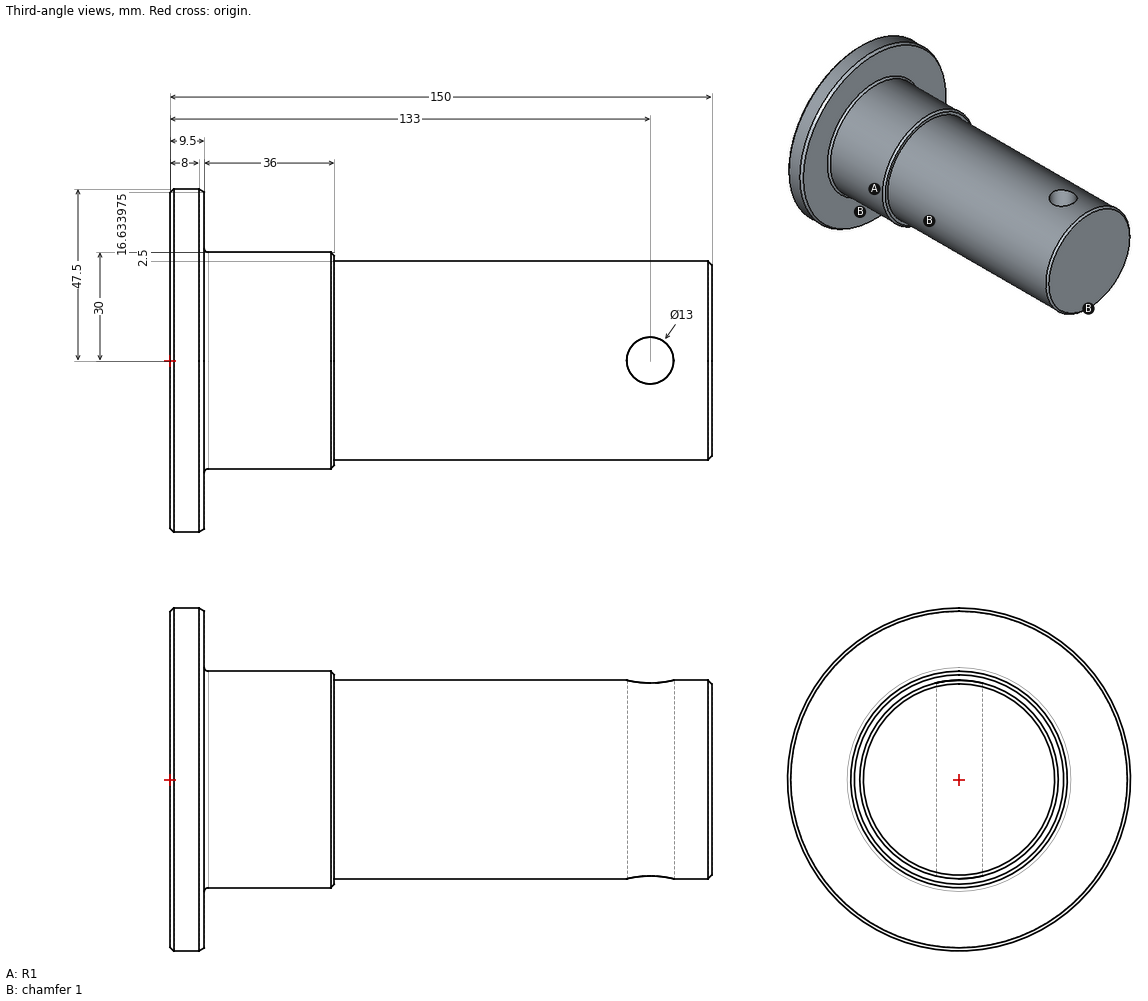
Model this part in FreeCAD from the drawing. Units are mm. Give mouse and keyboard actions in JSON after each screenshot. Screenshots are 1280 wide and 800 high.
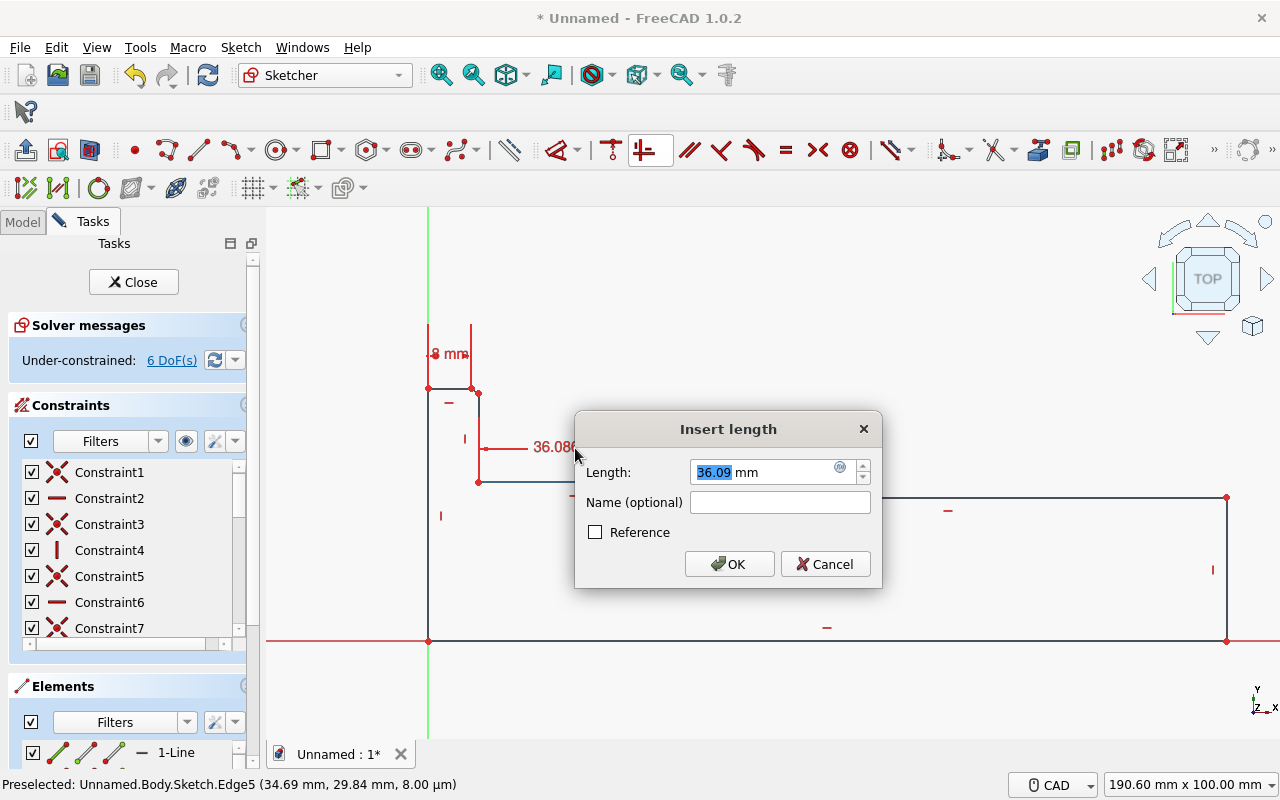
{"action": "type", "text": "36"}
{"action": "key", "text": "Return"}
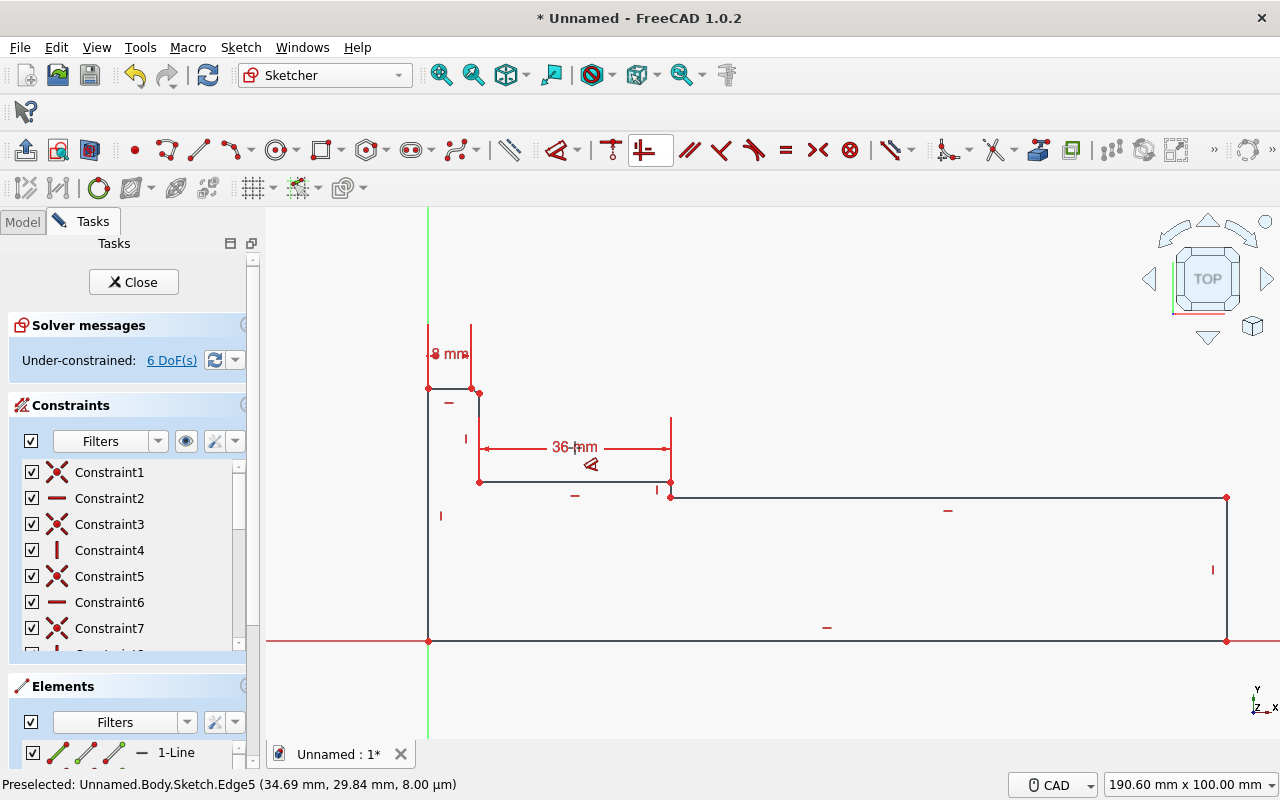
{"action": "left_click", "coordinate": [668, 641]}
{"action": "left_click", "coordinate": [772, 675]}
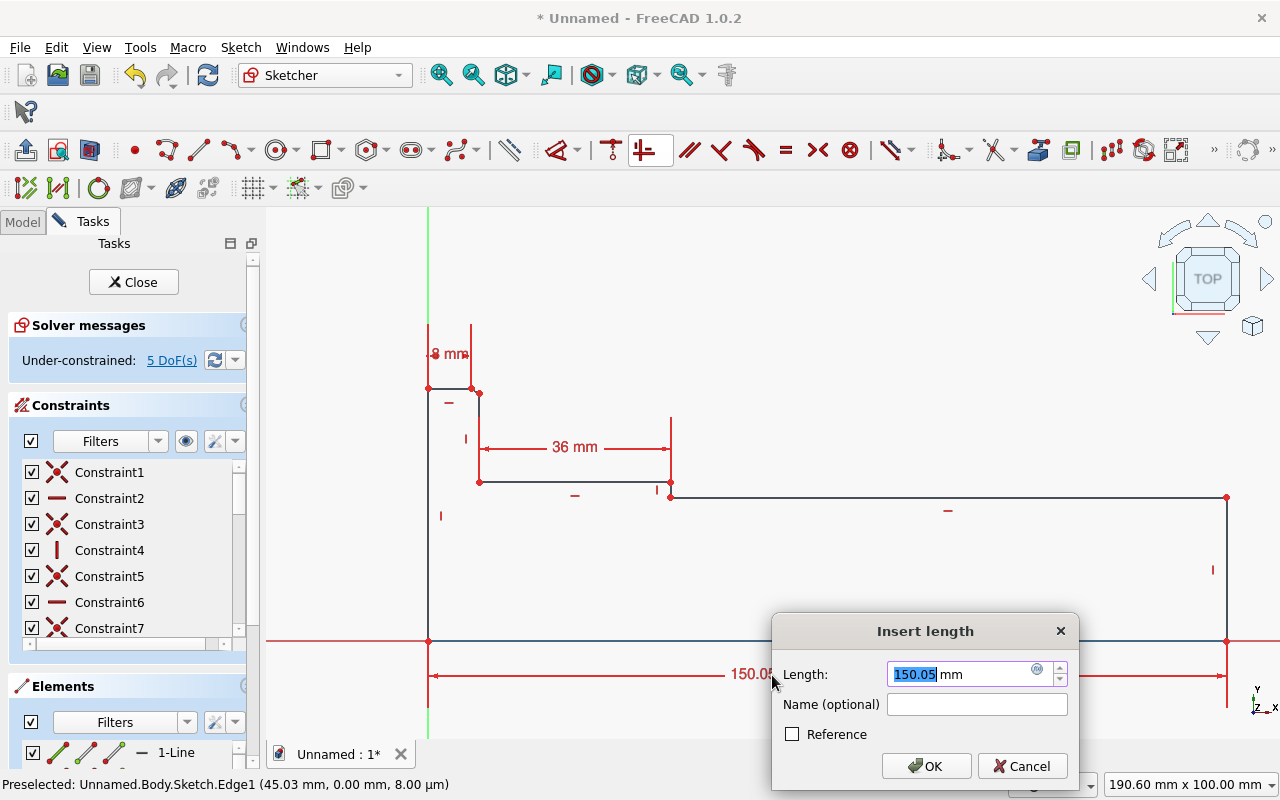
{"action": "type", "text": "150"}
{"action": "key", "text": "Return"}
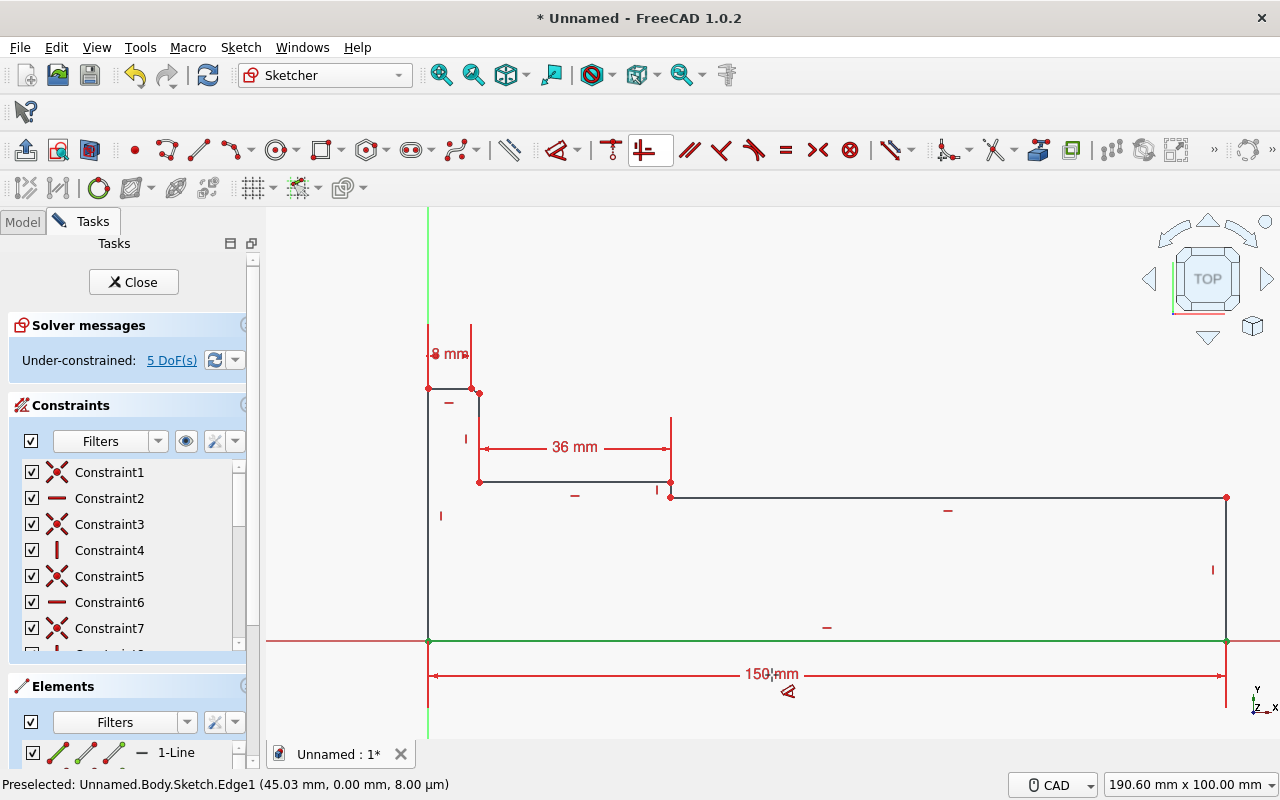
{"action": "scroll", "coordinate": [671, 490], "scroll_direction": "up", "scroll_amount": 6}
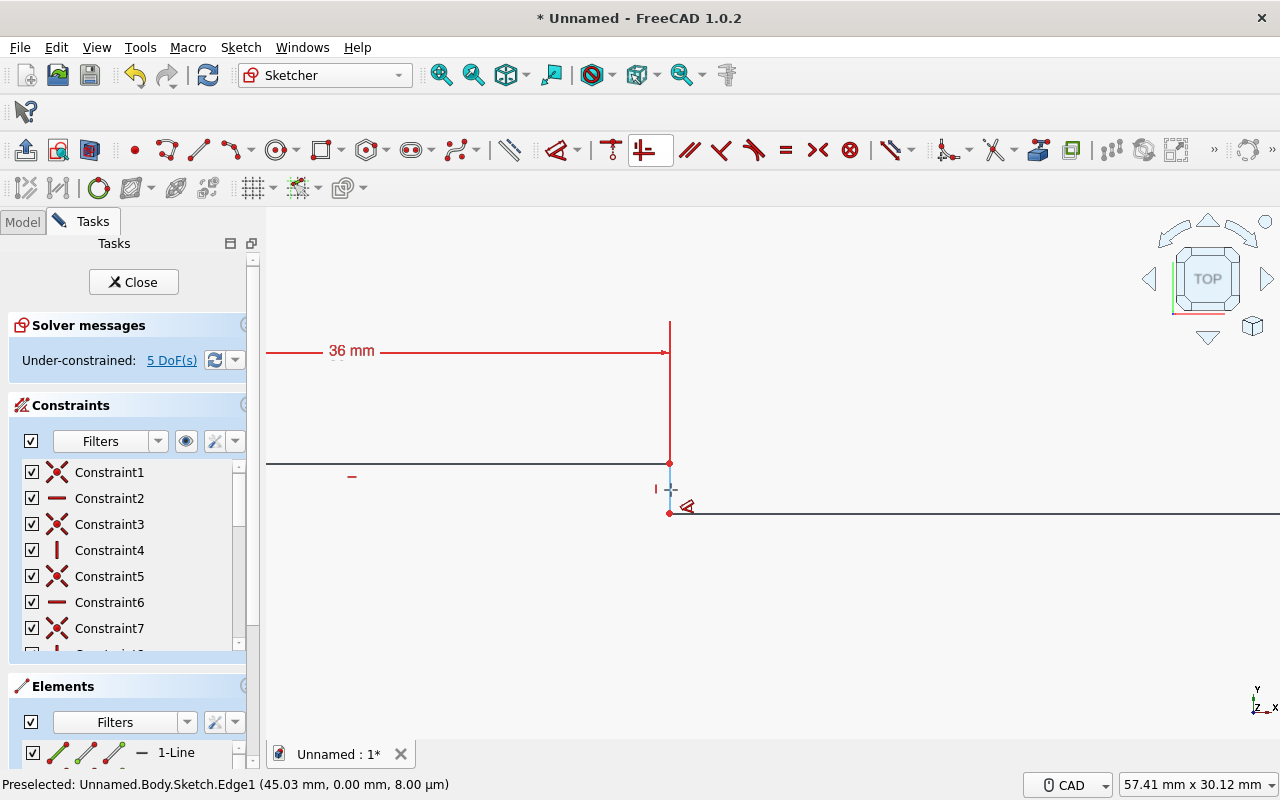
{"action": "left_click", "coordinate": [670, 489]}
{"action": "left_click", "coordinate": [636, 489]}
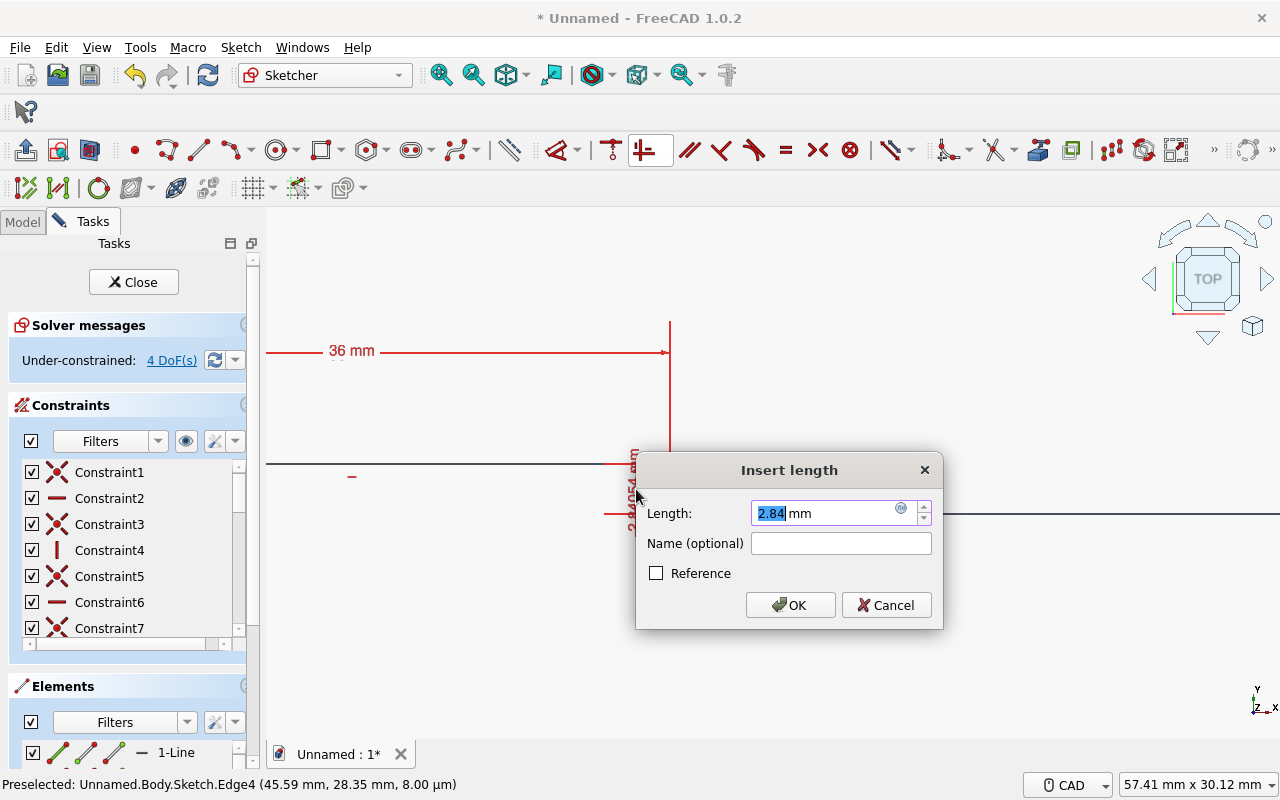
{"action": "type", "text": "2.5"}
{"action": "key", "text": "Return"}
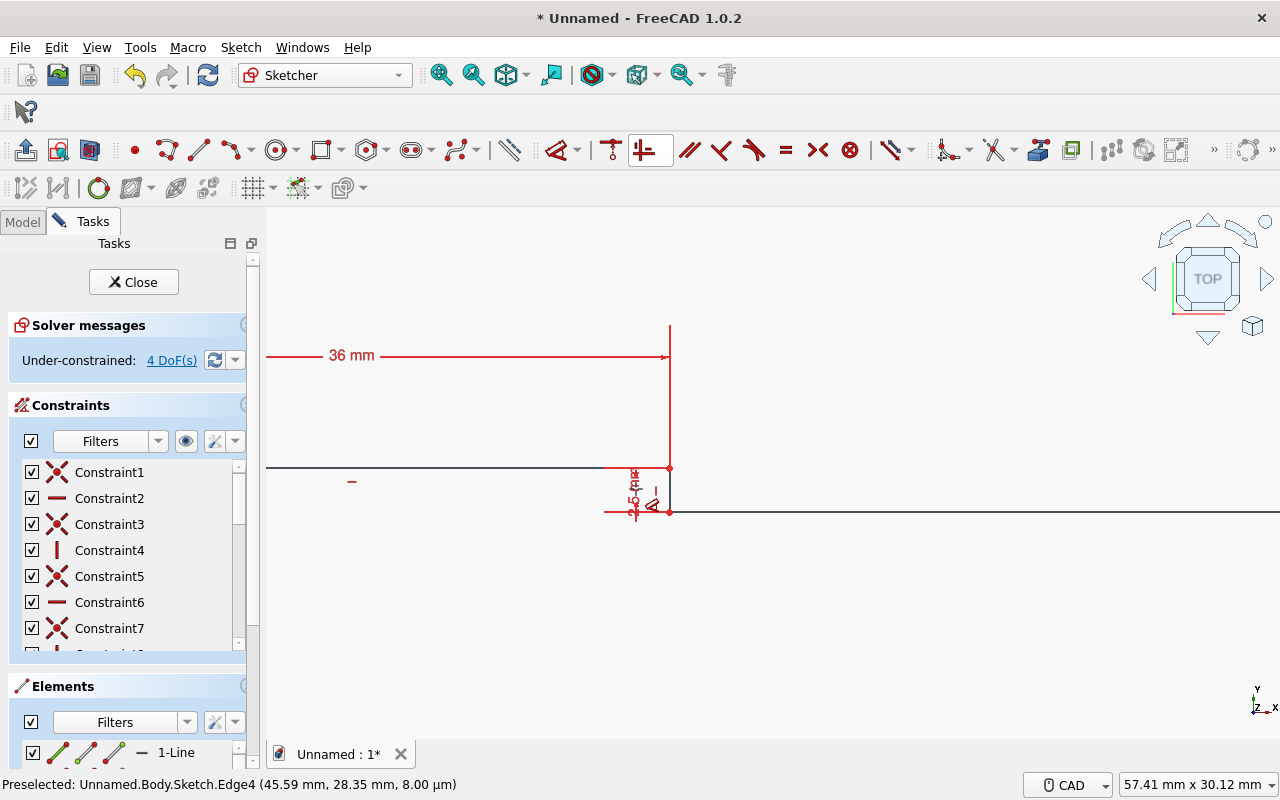
{"action": "scroll", "coordinate": [582, 448], "scroll_direction": "down", "scroll_amount": 8}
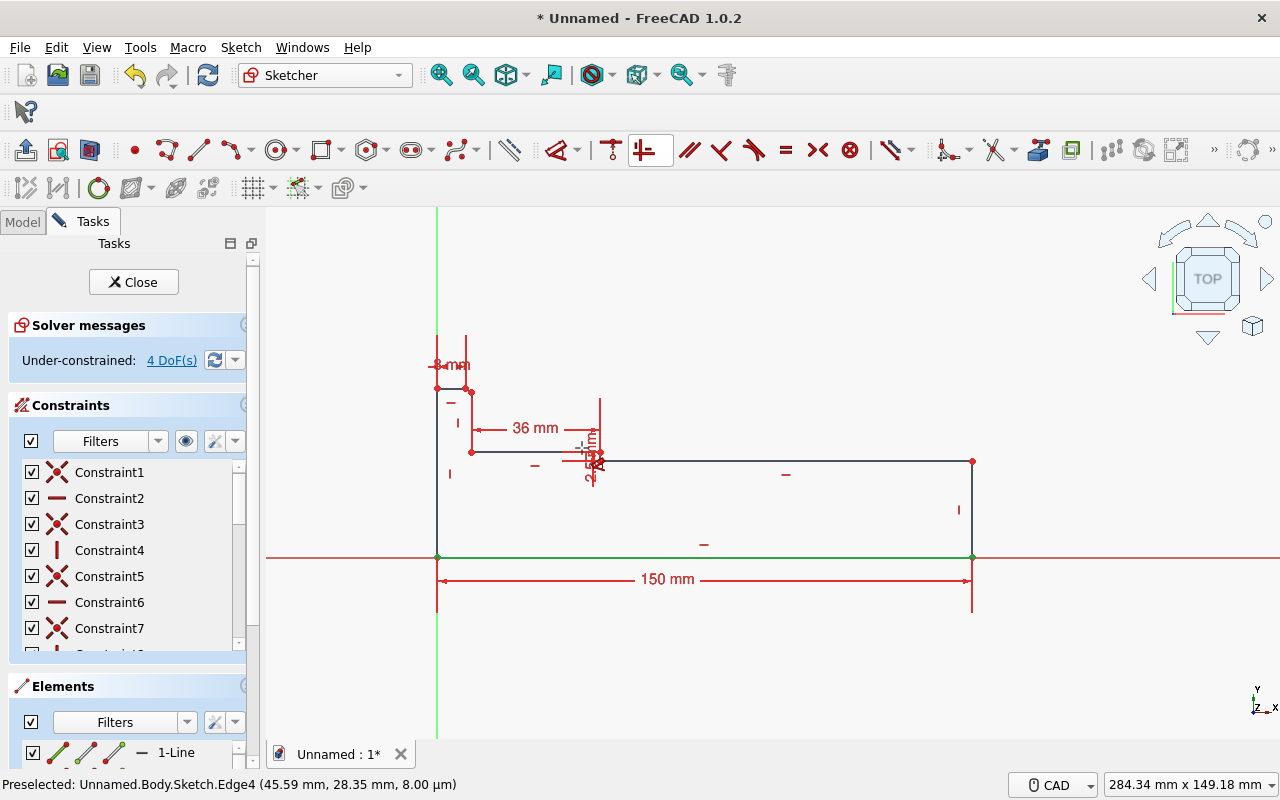
{"action": "scroll", "coordinate": [600, 452], "scroll_direction": "up", "scroll_amount": 2}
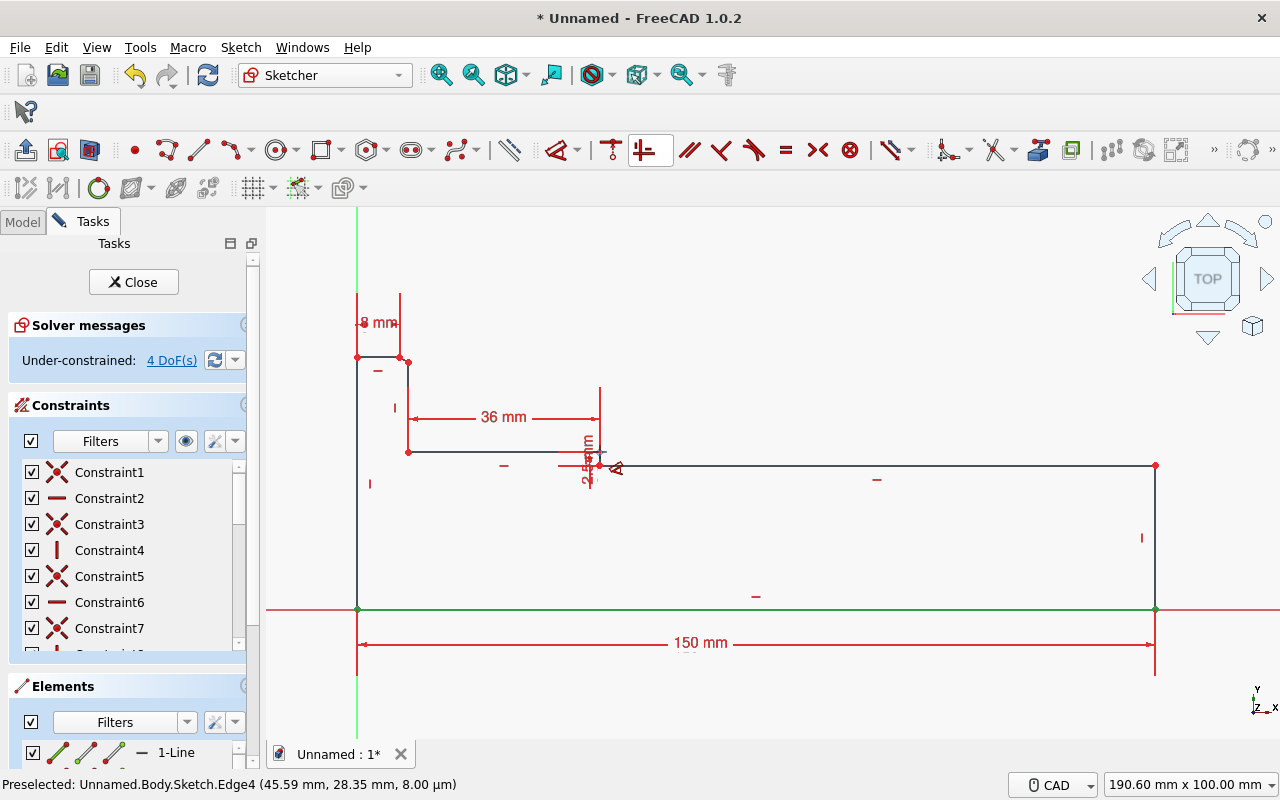
{"action": "left_click", "coordinate": [600, 452]}
{"action": "left_click", "coordinate": [323, 531]}